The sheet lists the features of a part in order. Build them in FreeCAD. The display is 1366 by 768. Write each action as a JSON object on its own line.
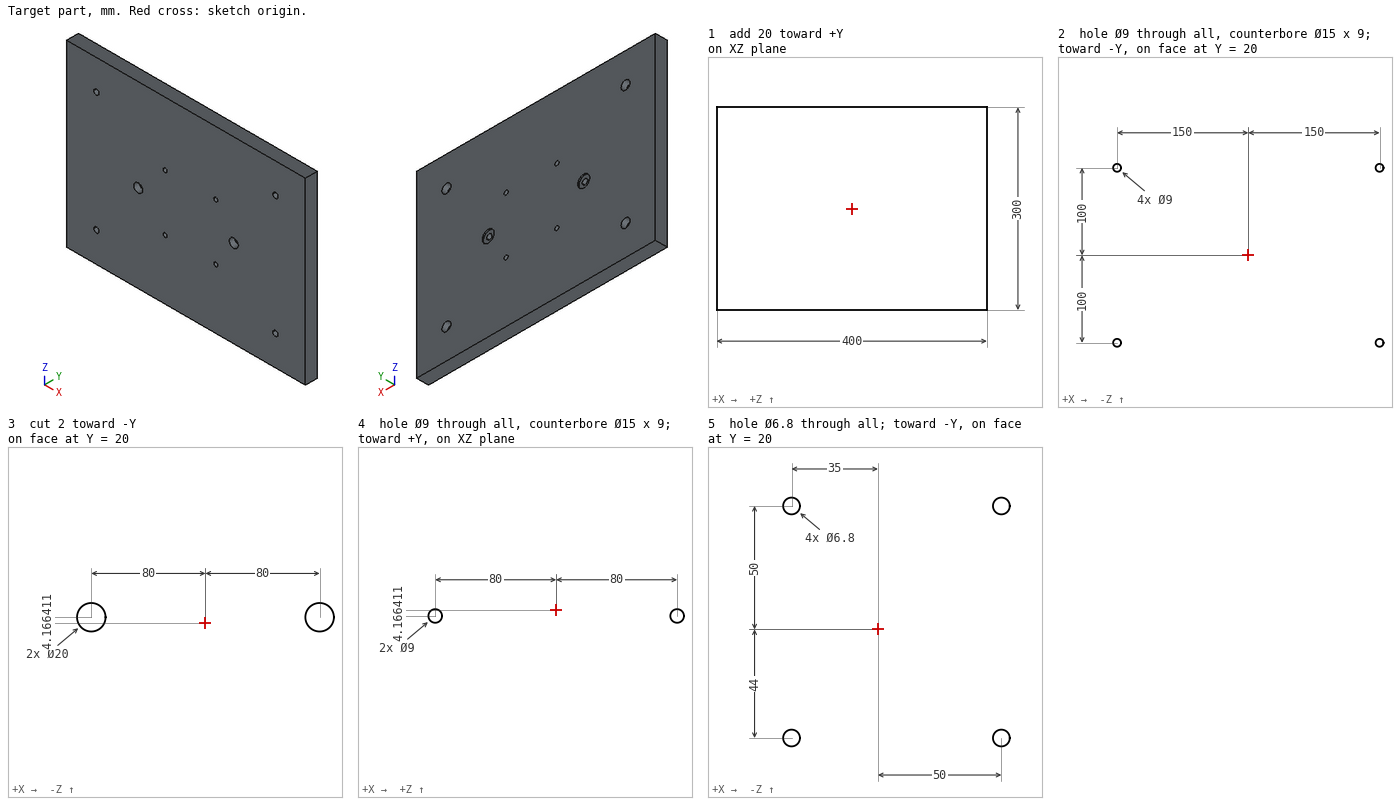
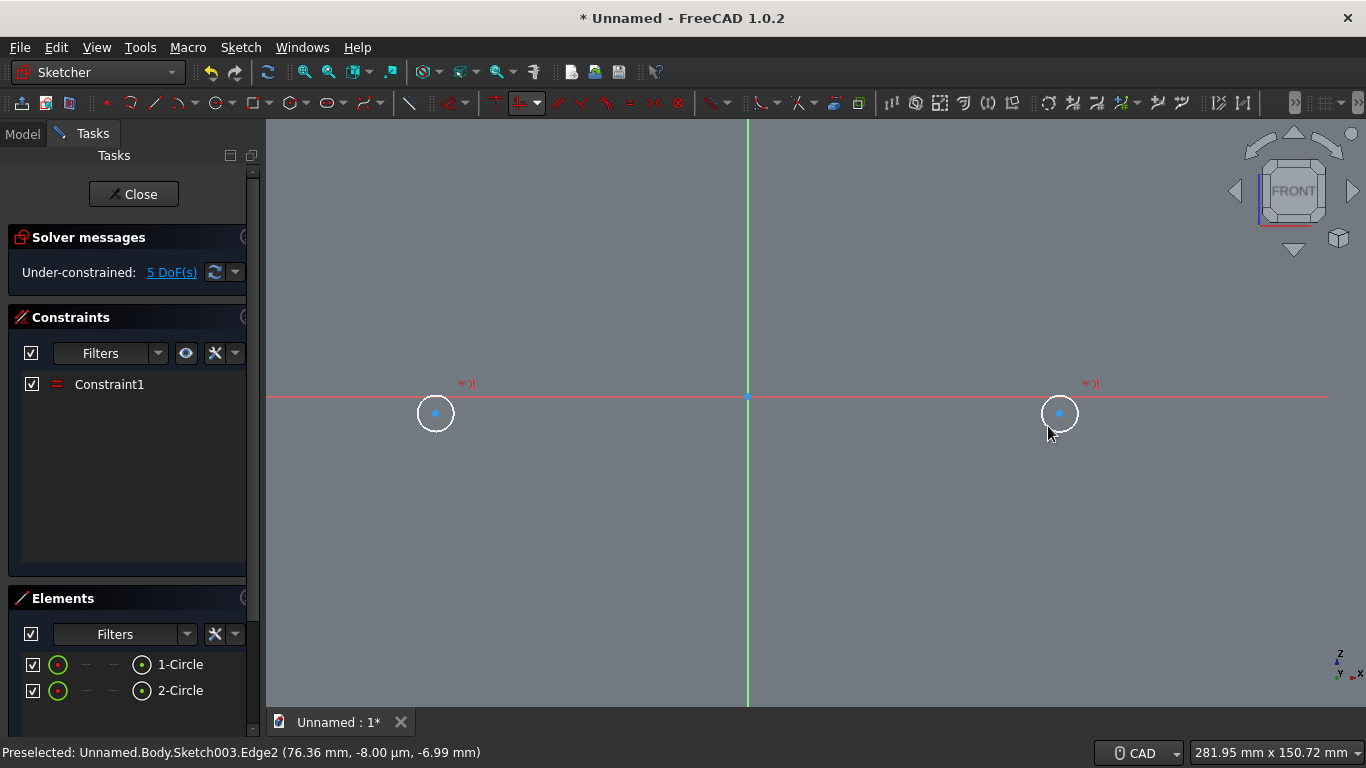
{"action": "left_click", "coordinate": [436, 413]}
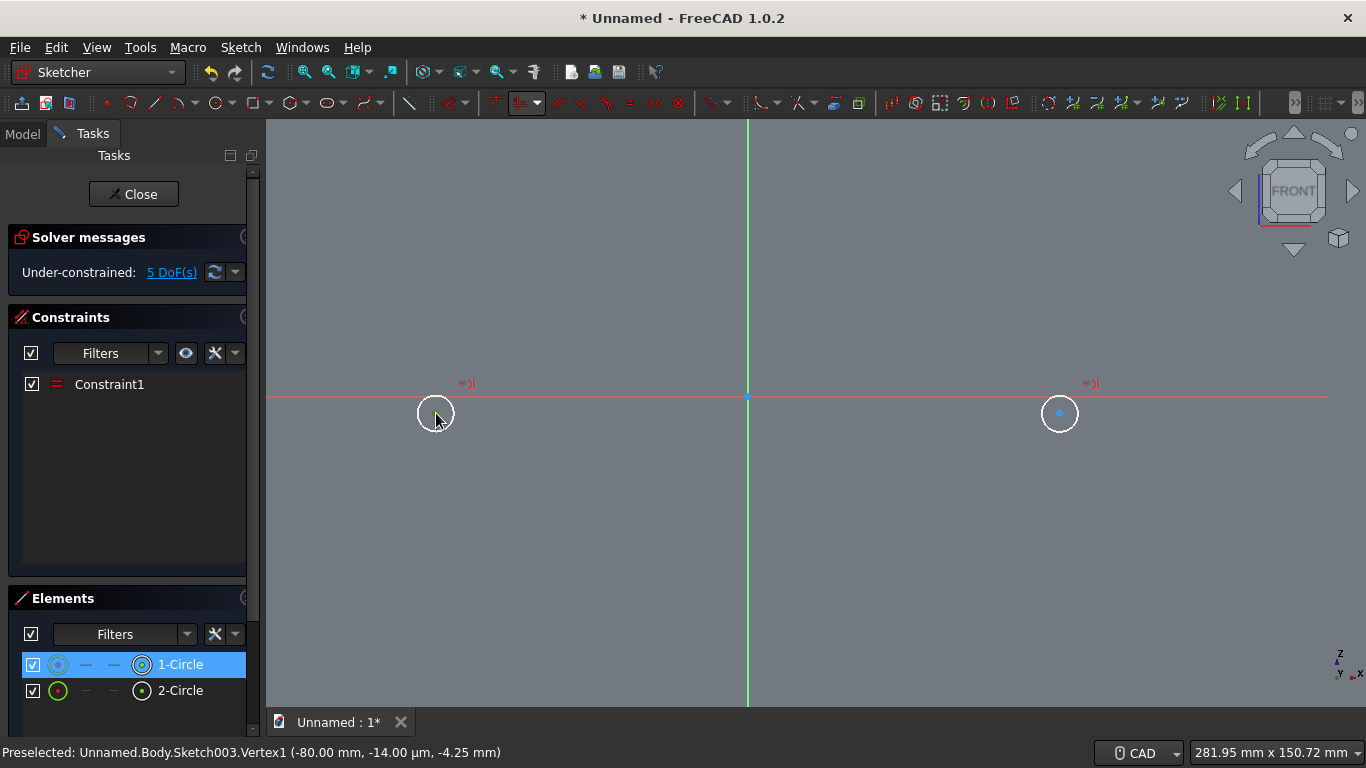
{"action": "left_click", "coordinate": [1060, 414]}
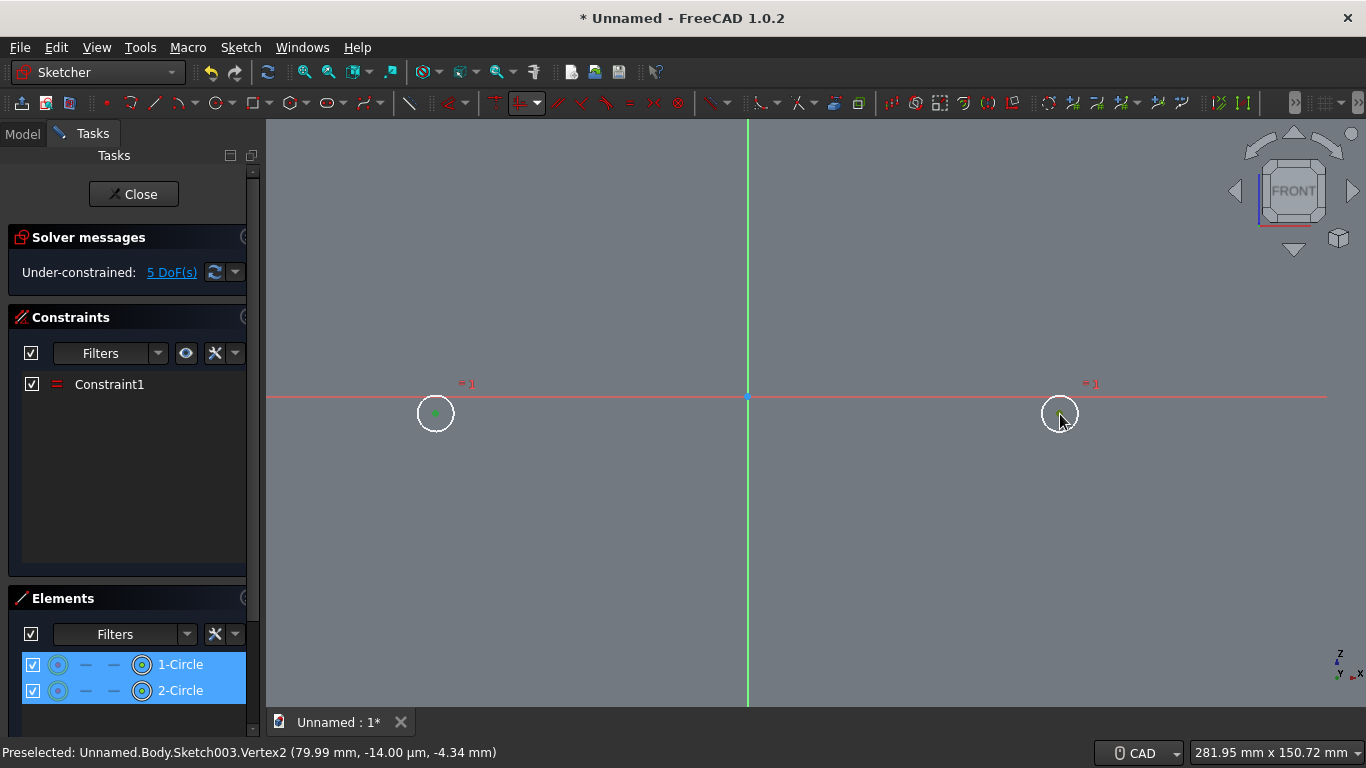
{"action": "key", "text": "h"}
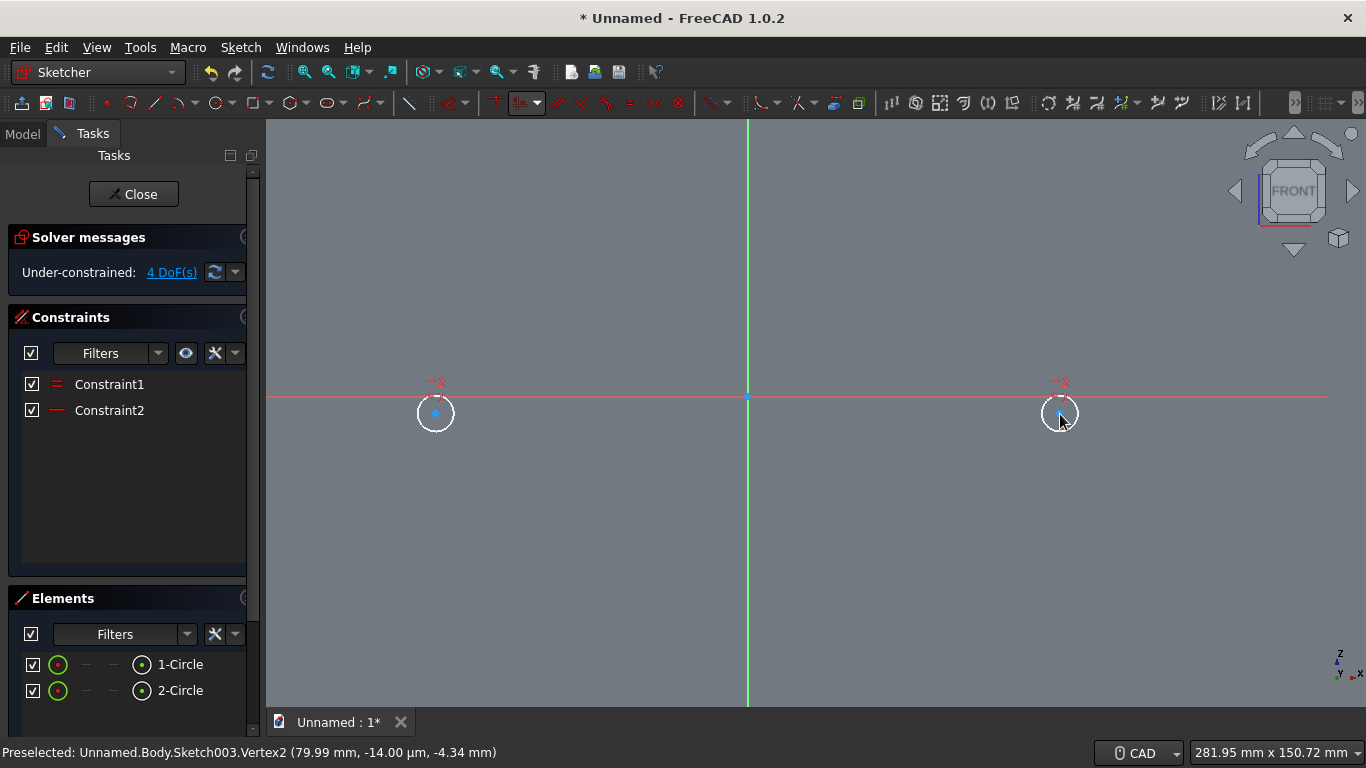
{"action": "left_click", "coordinate": [448, 104]}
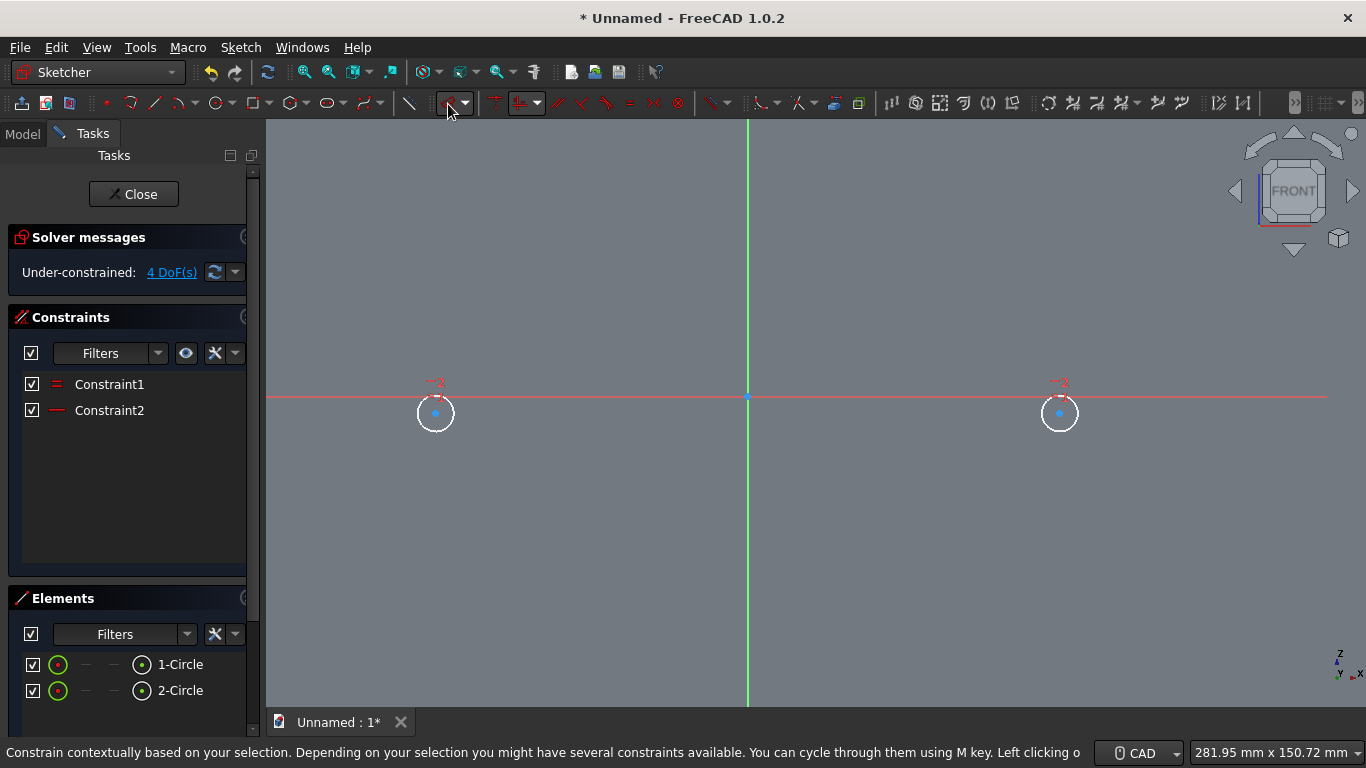
{"action": "left_click", "coordinate": [448, 401]}
{"action": "left_click", "coordinate": [470, 378]}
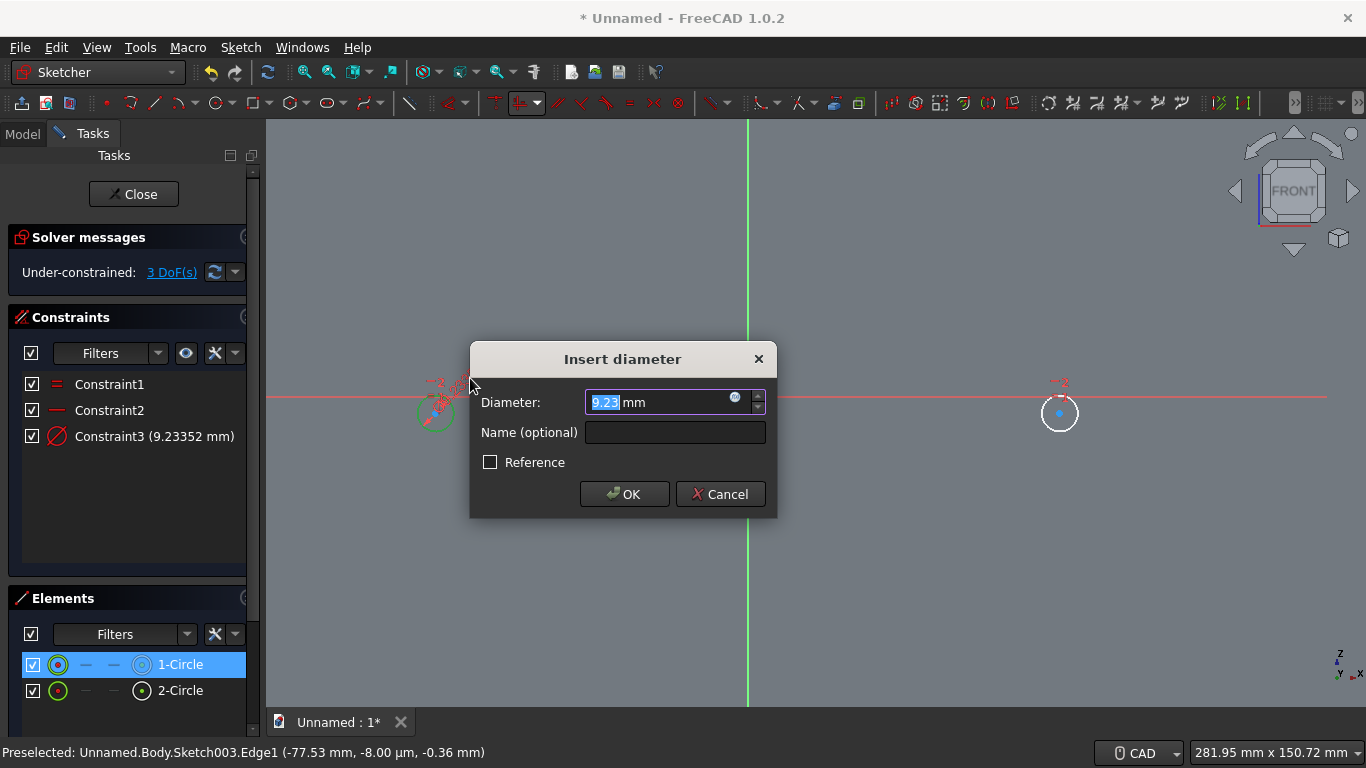
{"action": "type", "text": "9"}
{"action": "key", "text": "Return"}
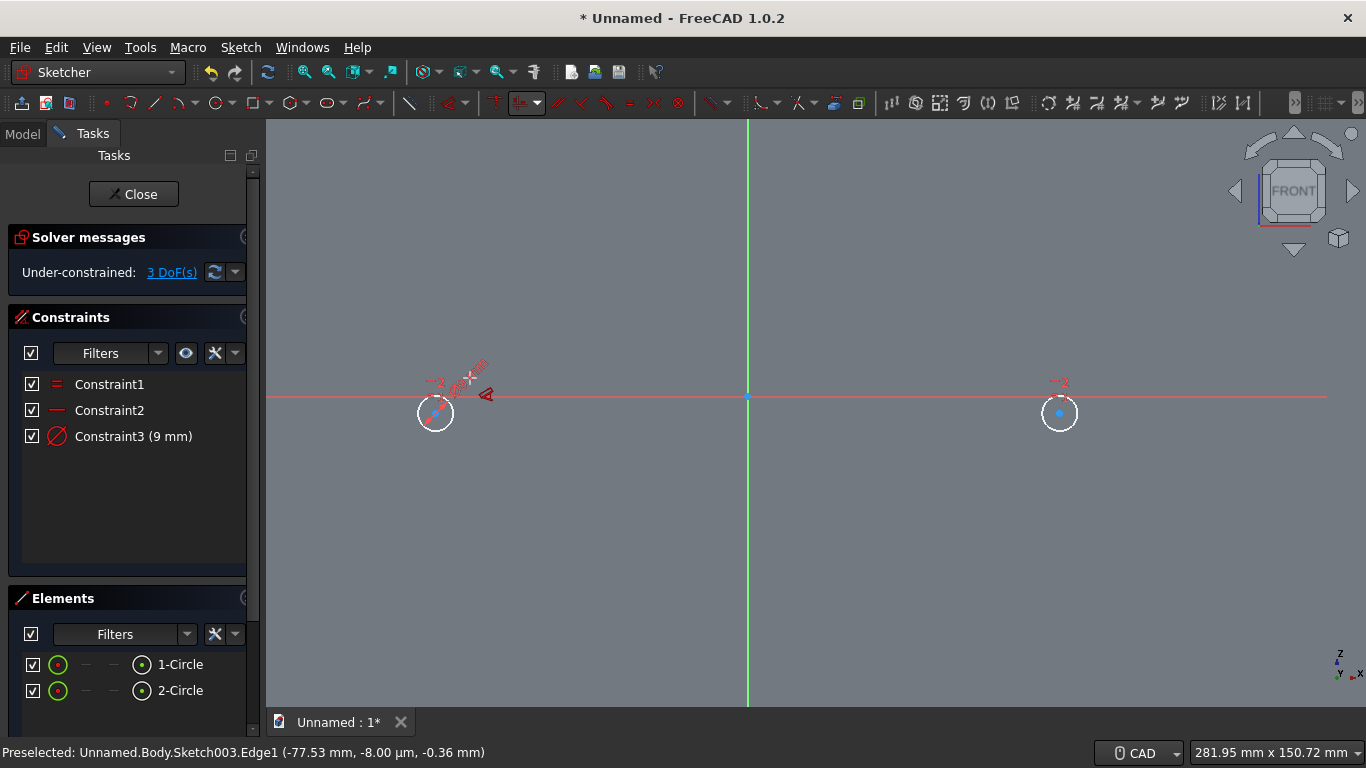
{"action": "left_click", "coordinate": [436, 413]}
{"action": "left_click", "coordinate": [592, 363]}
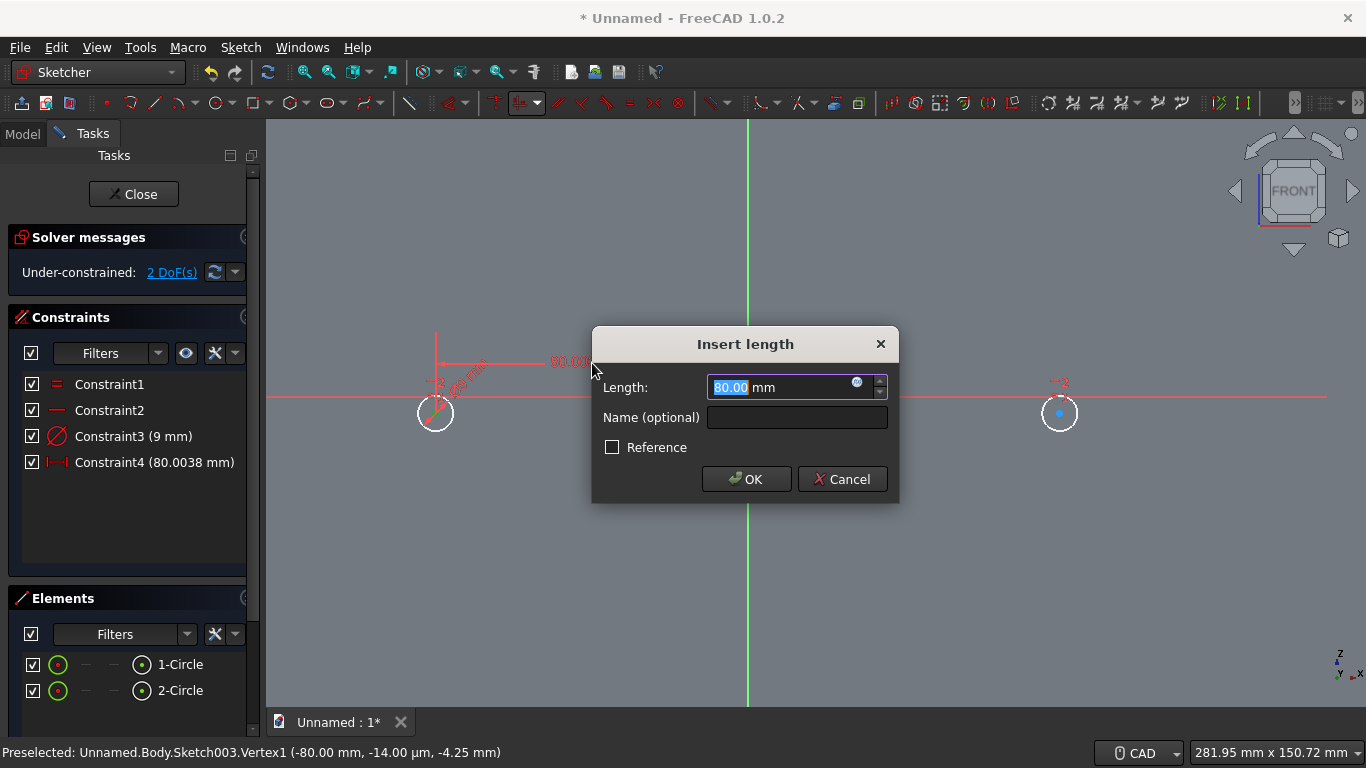
{"action": "type", "text": "80"}
{"action": "key", "text": "Return"}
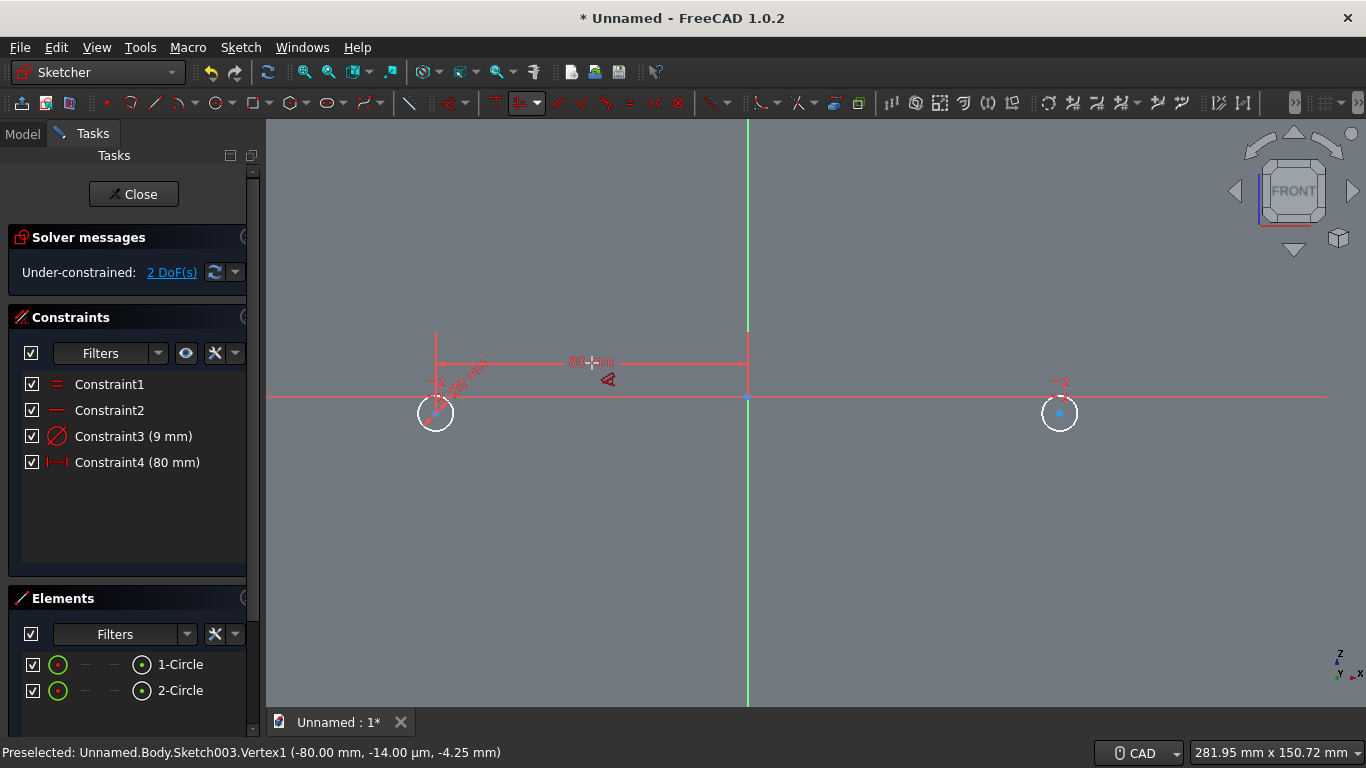
{"action": "left_click", "coordinate": [1060, 413]}
{"action": "left_click", "coordinate": [904, 363]}